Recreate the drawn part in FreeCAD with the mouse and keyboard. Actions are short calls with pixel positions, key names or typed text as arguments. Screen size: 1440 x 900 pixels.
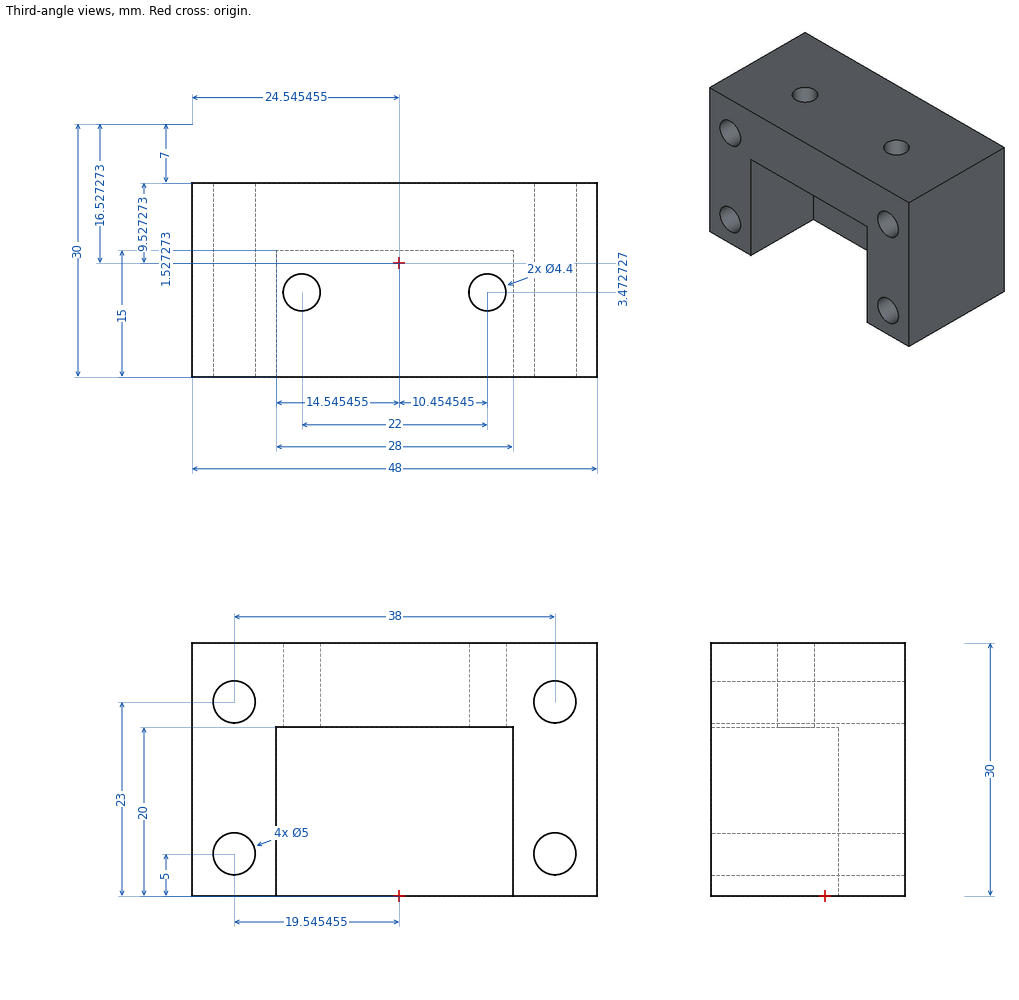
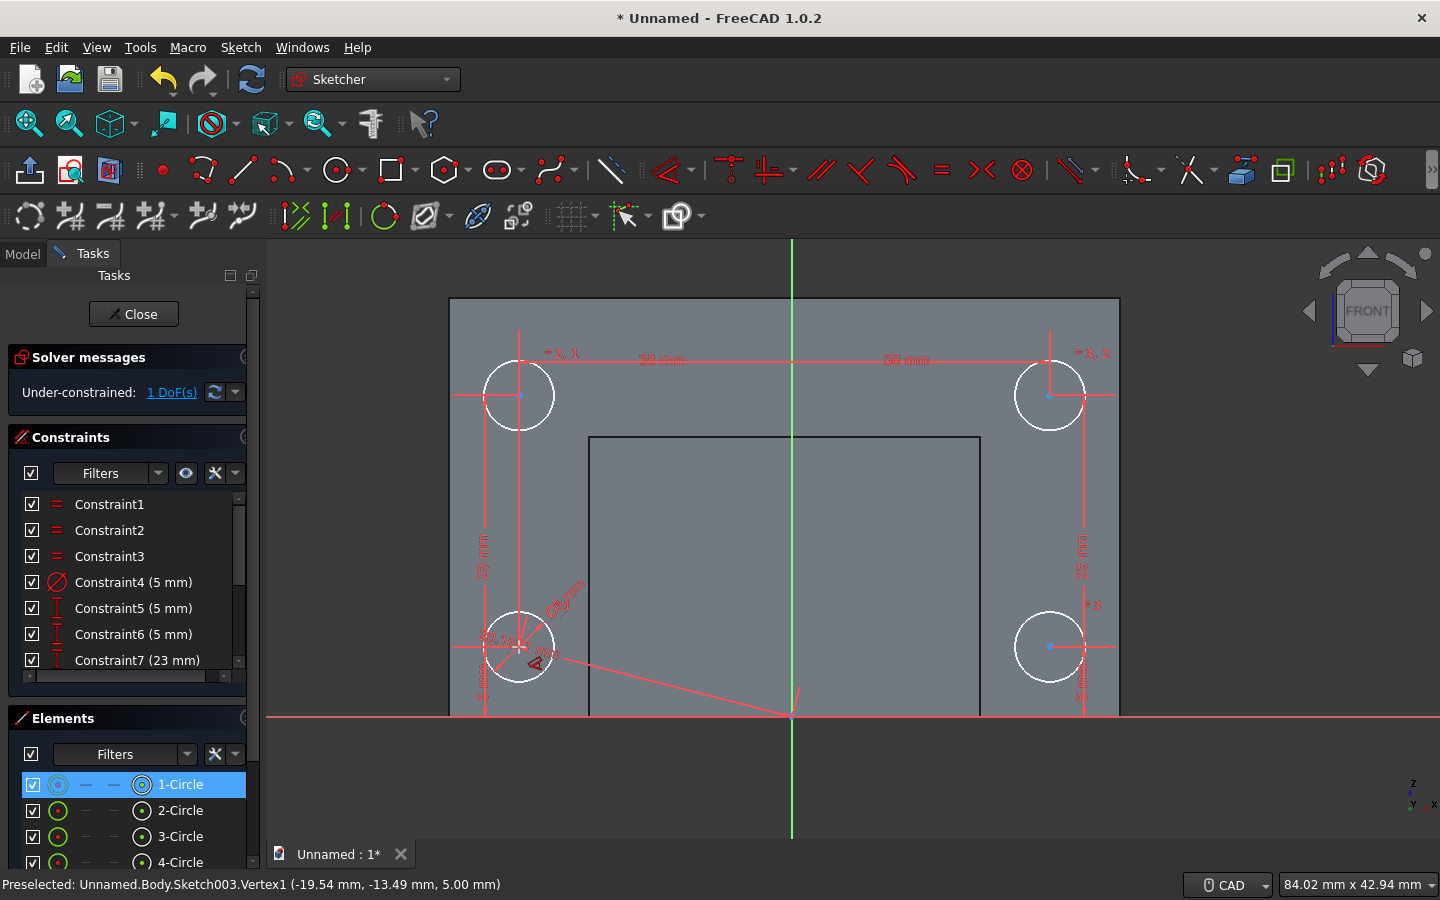
click(1050, 647)
click(662, 681)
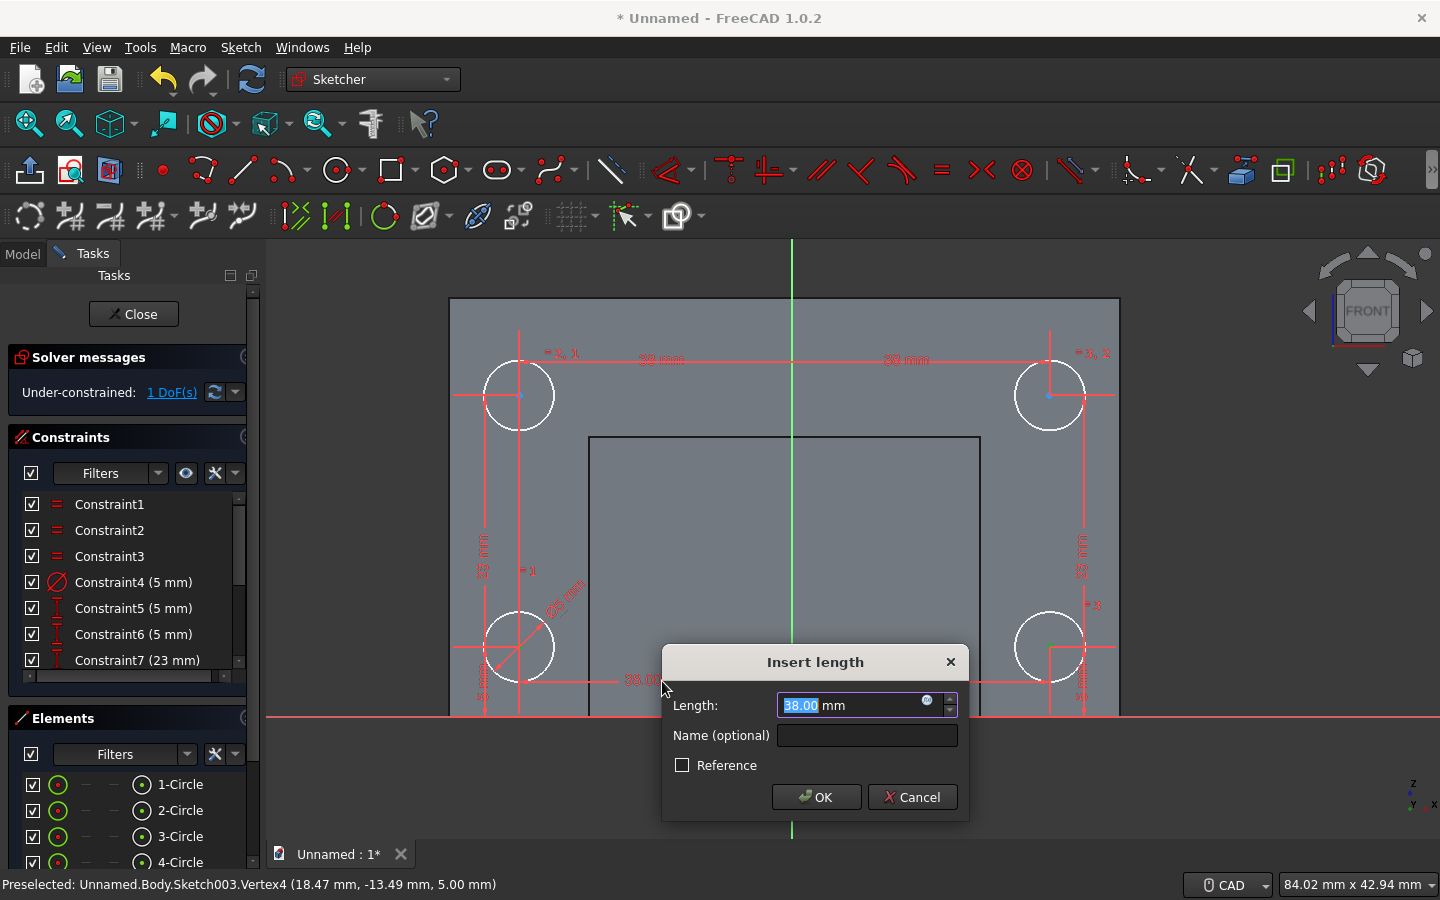
text(38)
key(Return)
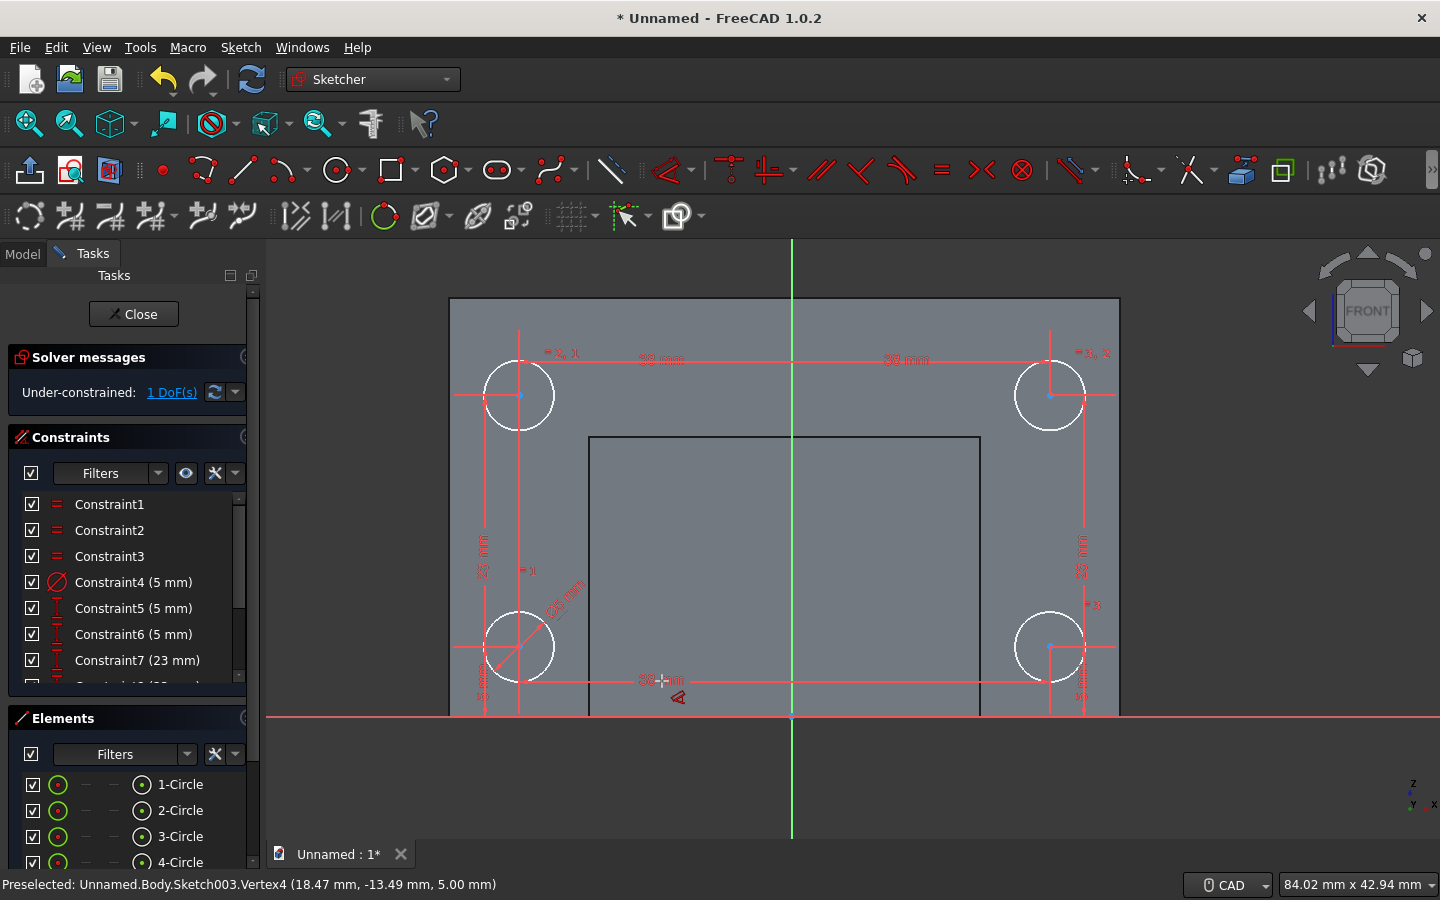
click(519, 647)
click(656, 751)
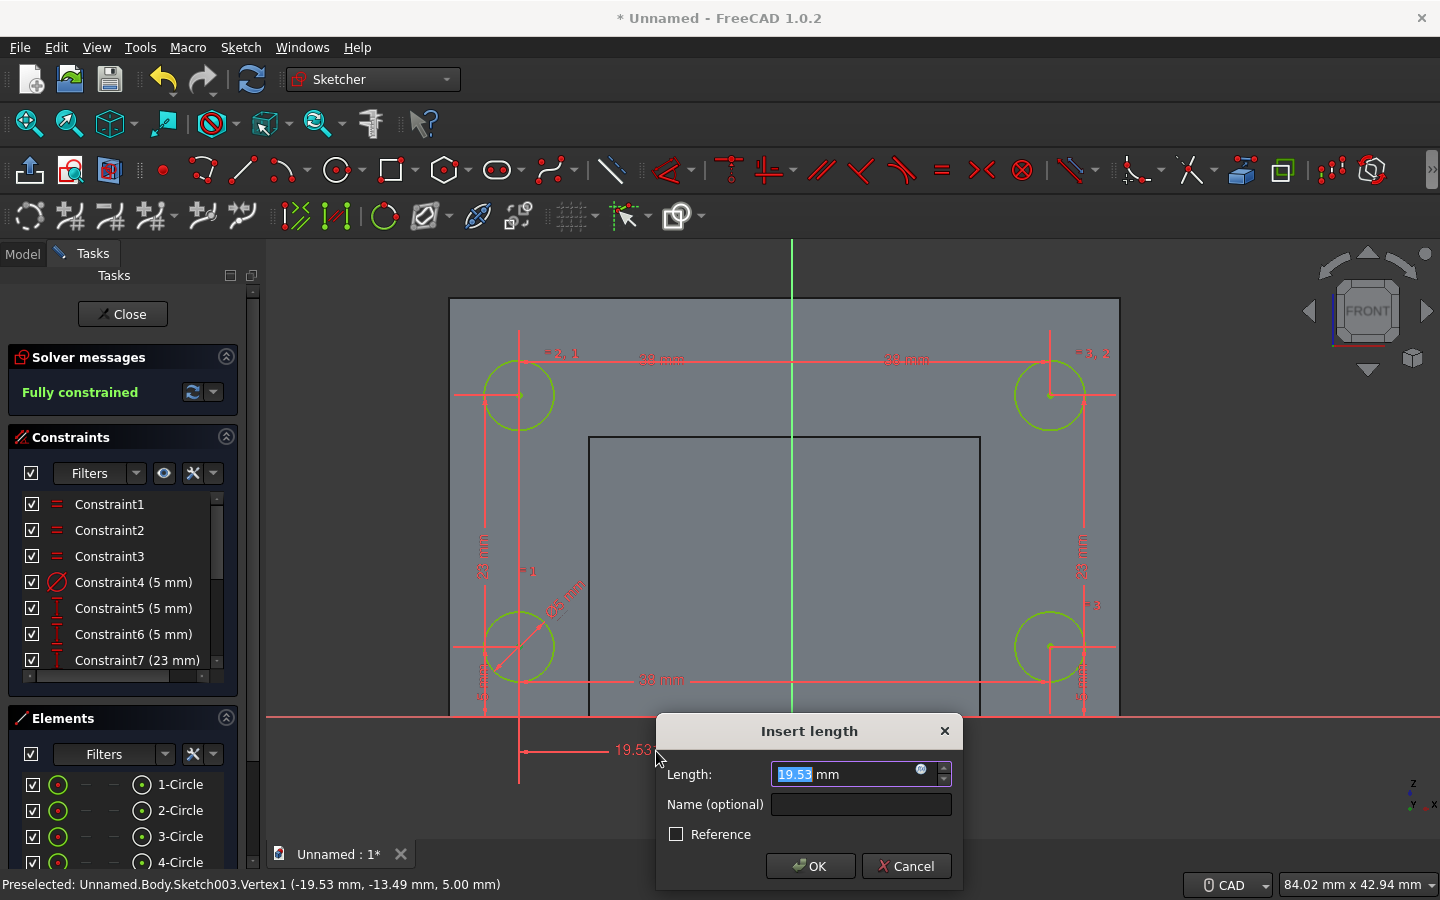
text(19.545455)
key(Return)
key(Escape)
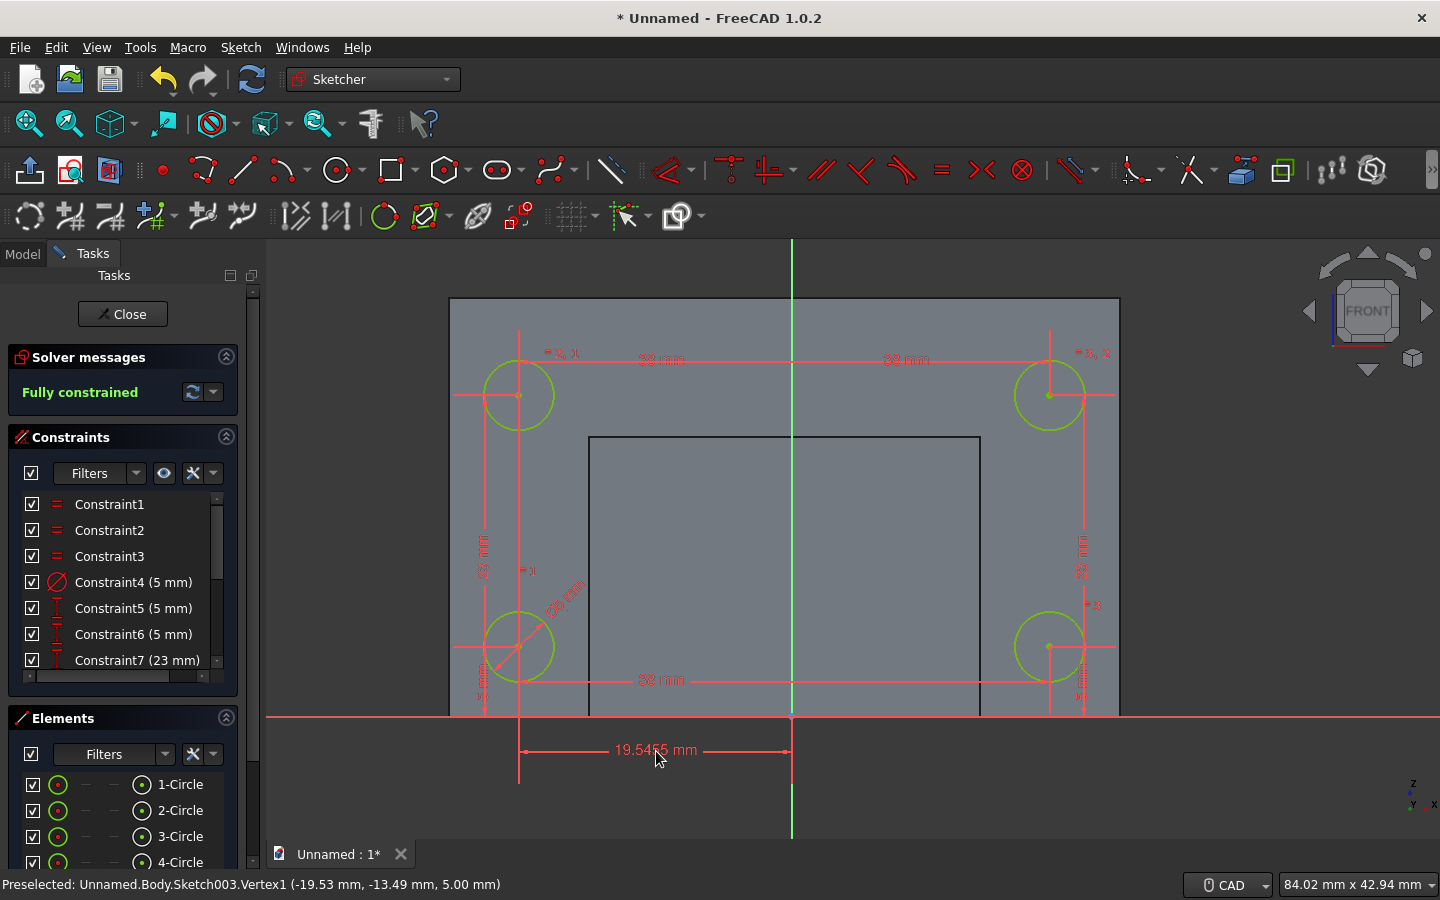
click(123, 314)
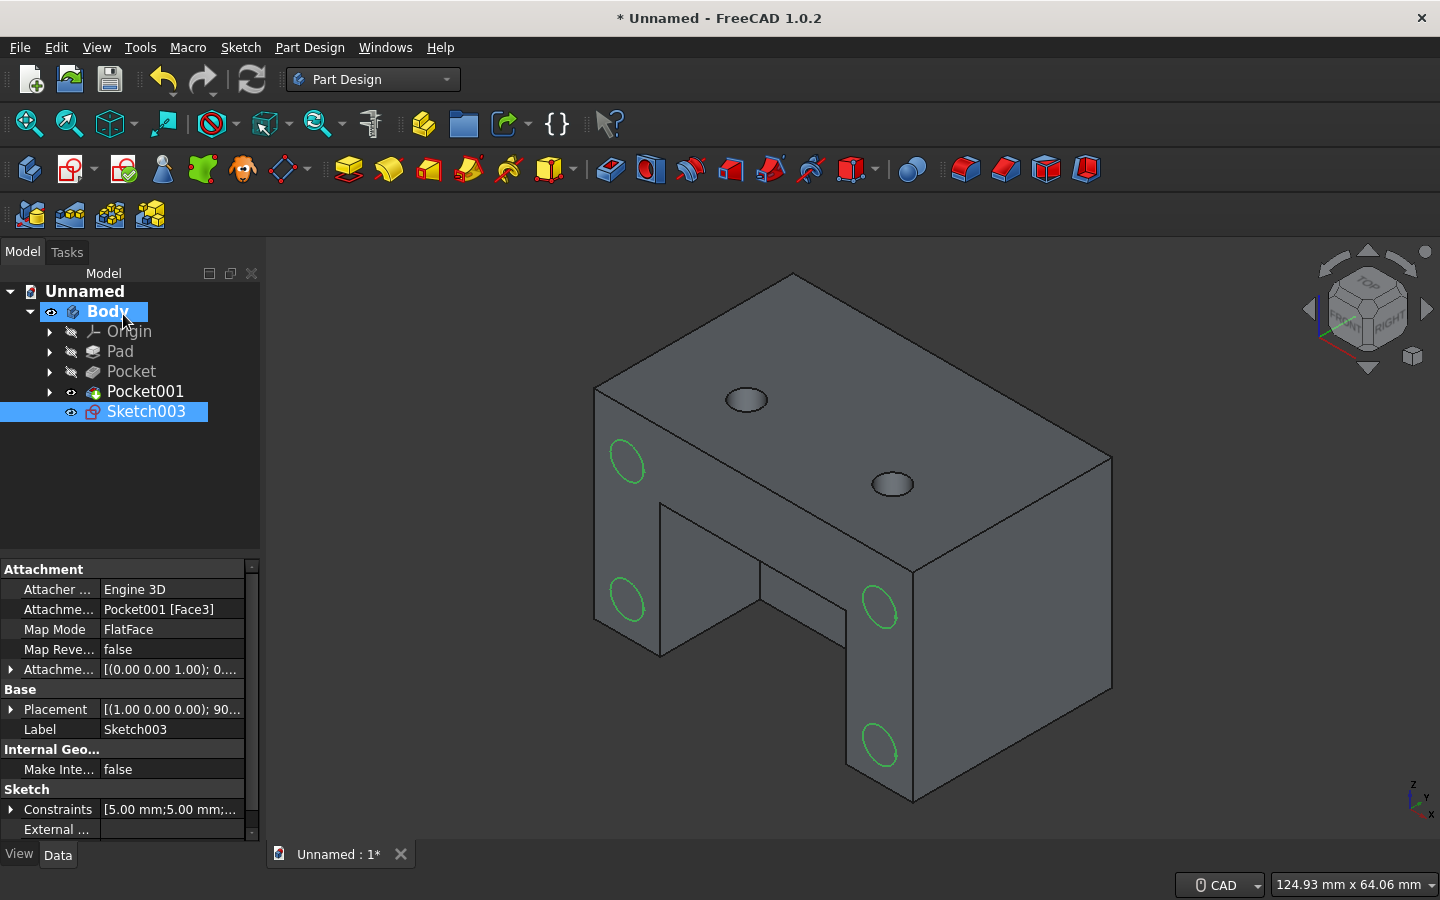
click(612, 170)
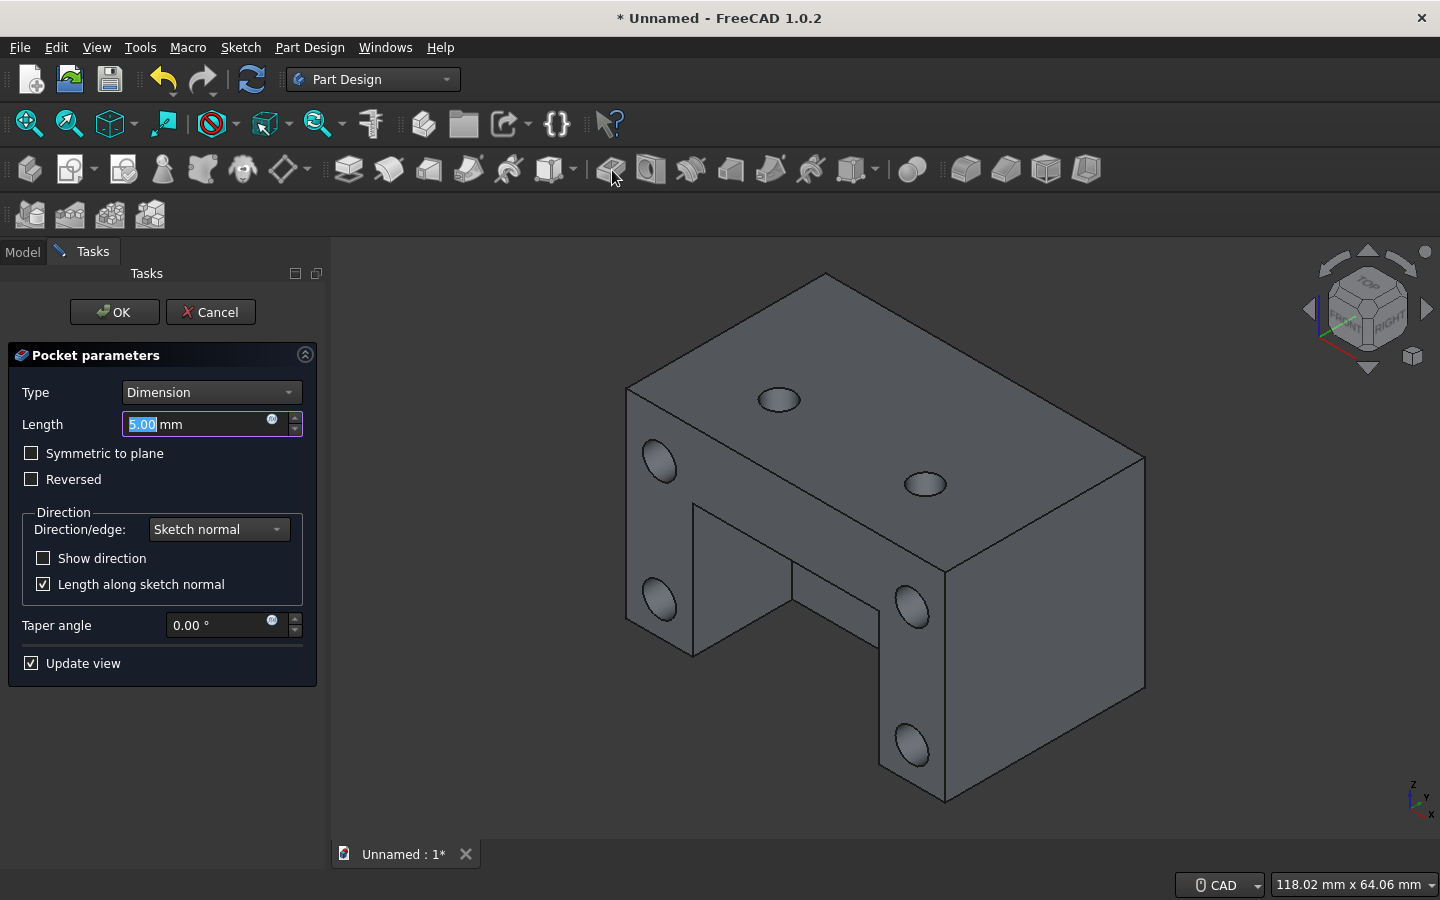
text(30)
key(Tab)